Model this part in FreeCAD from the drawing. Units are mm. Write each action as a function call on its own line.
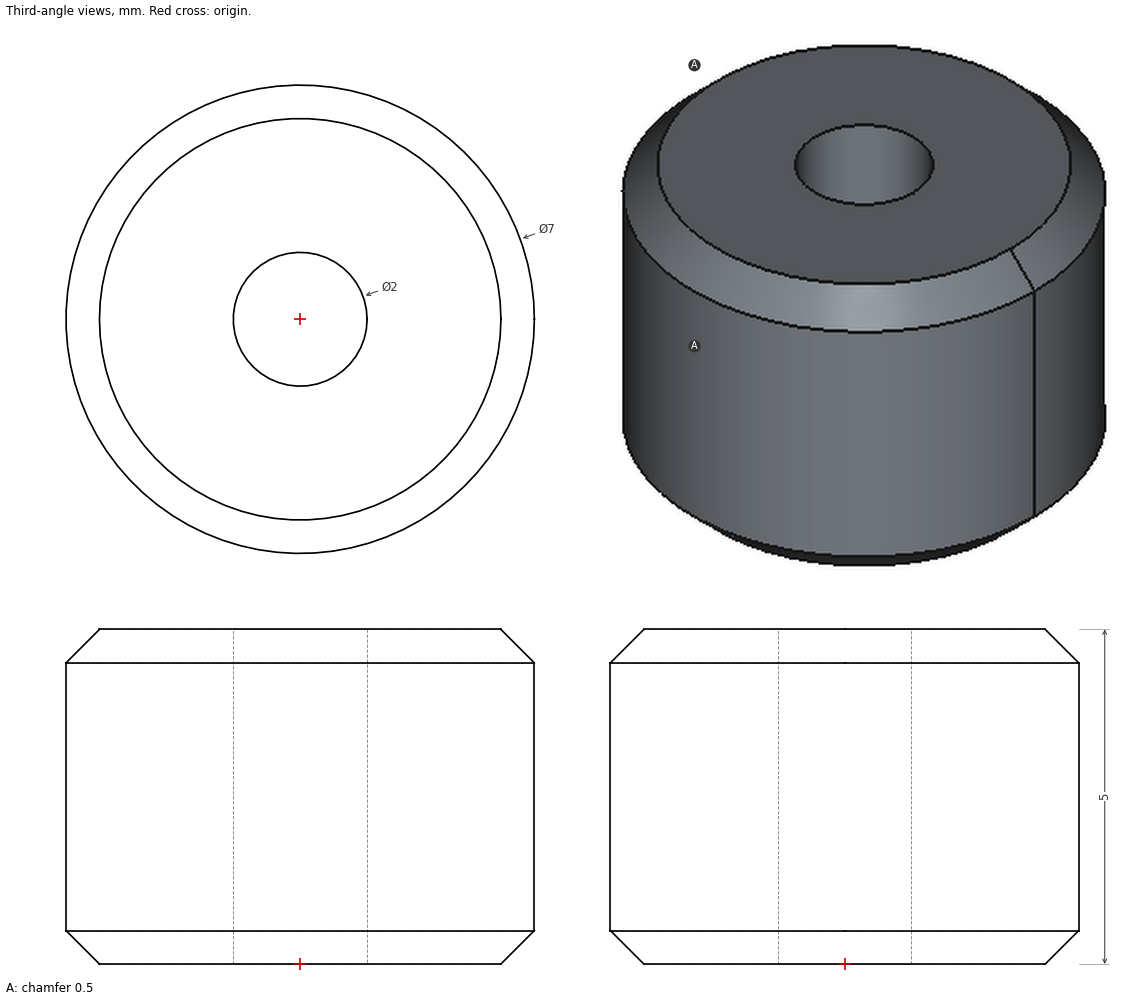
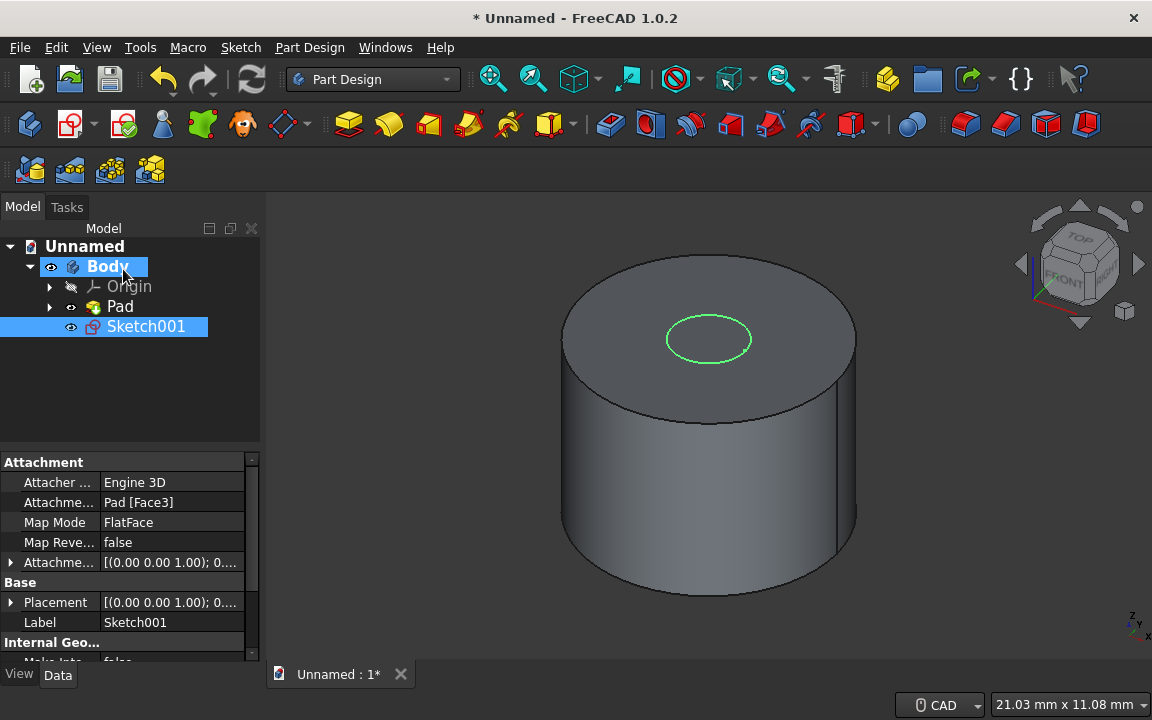
click(612, 124)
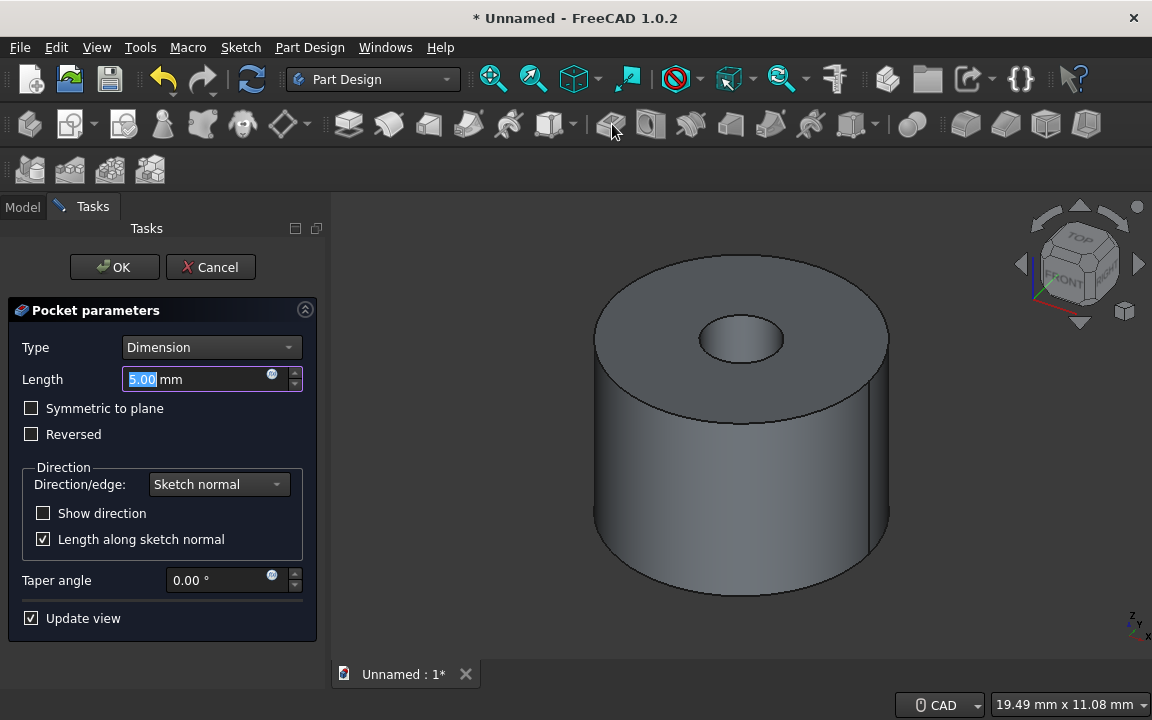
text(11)
key(Tab)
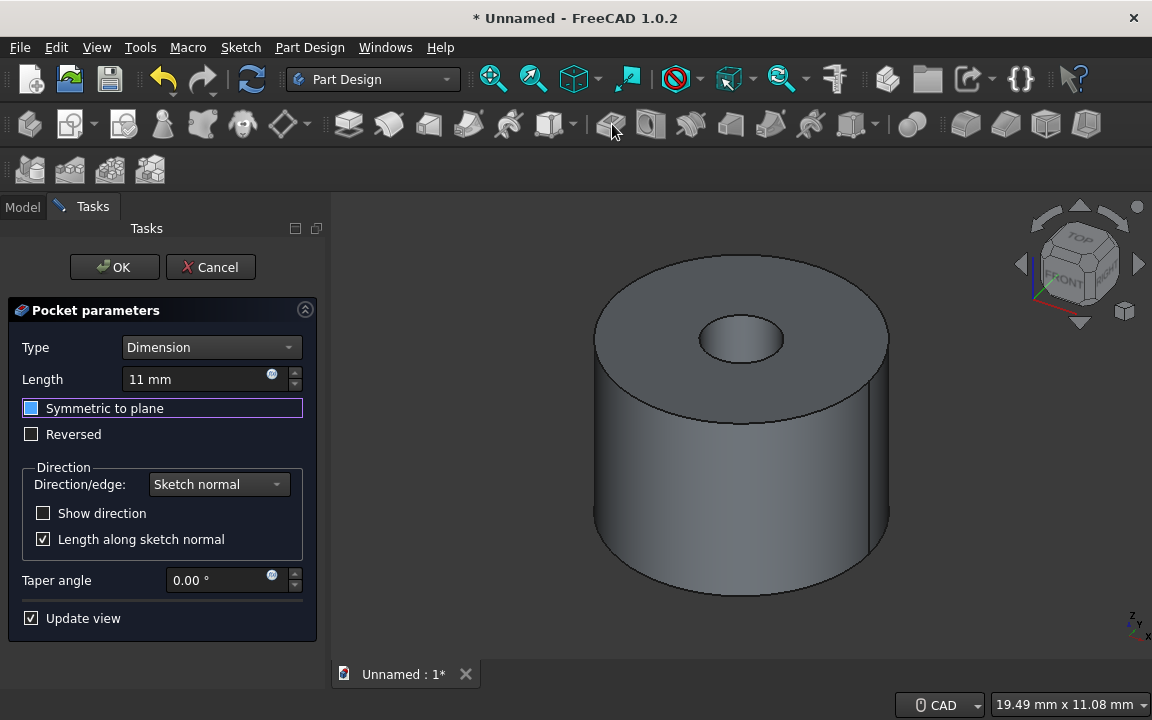
click(115, 267)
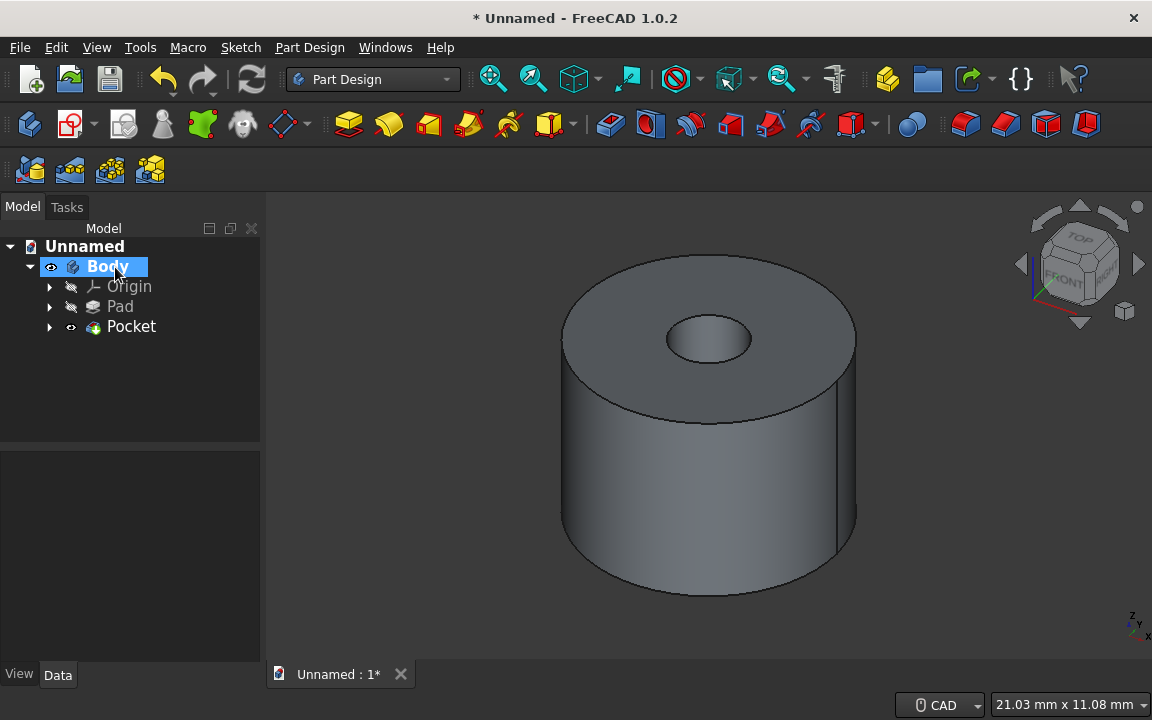
click(562, 347)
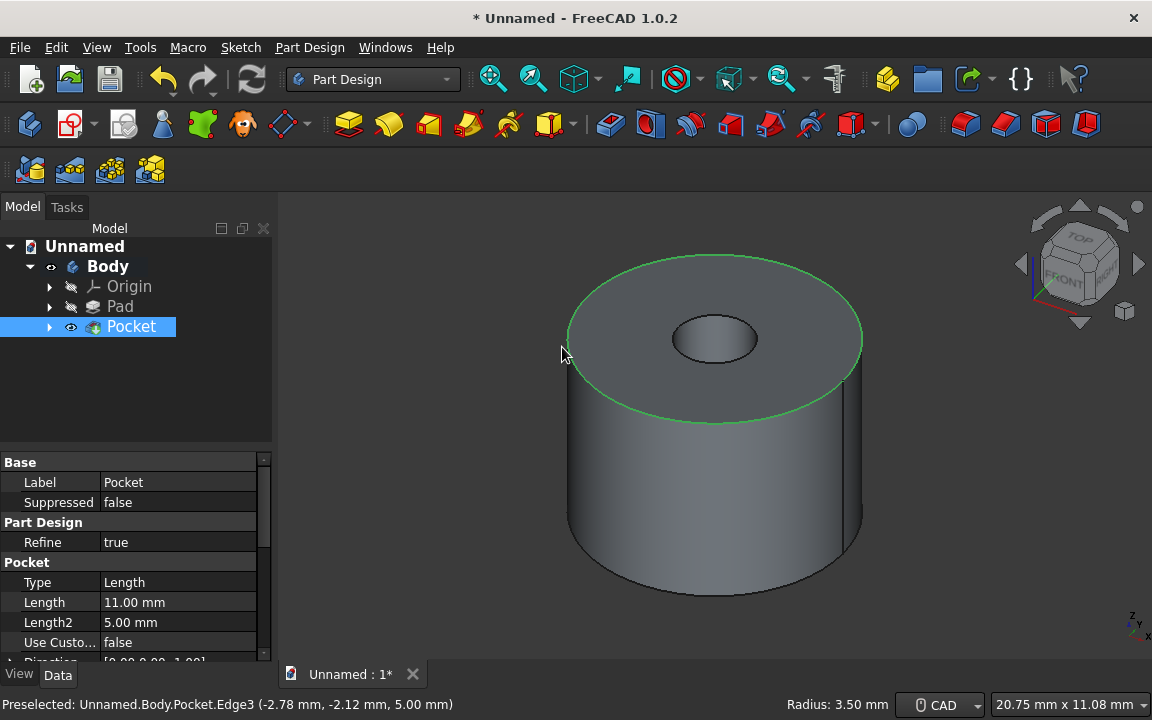
key(0)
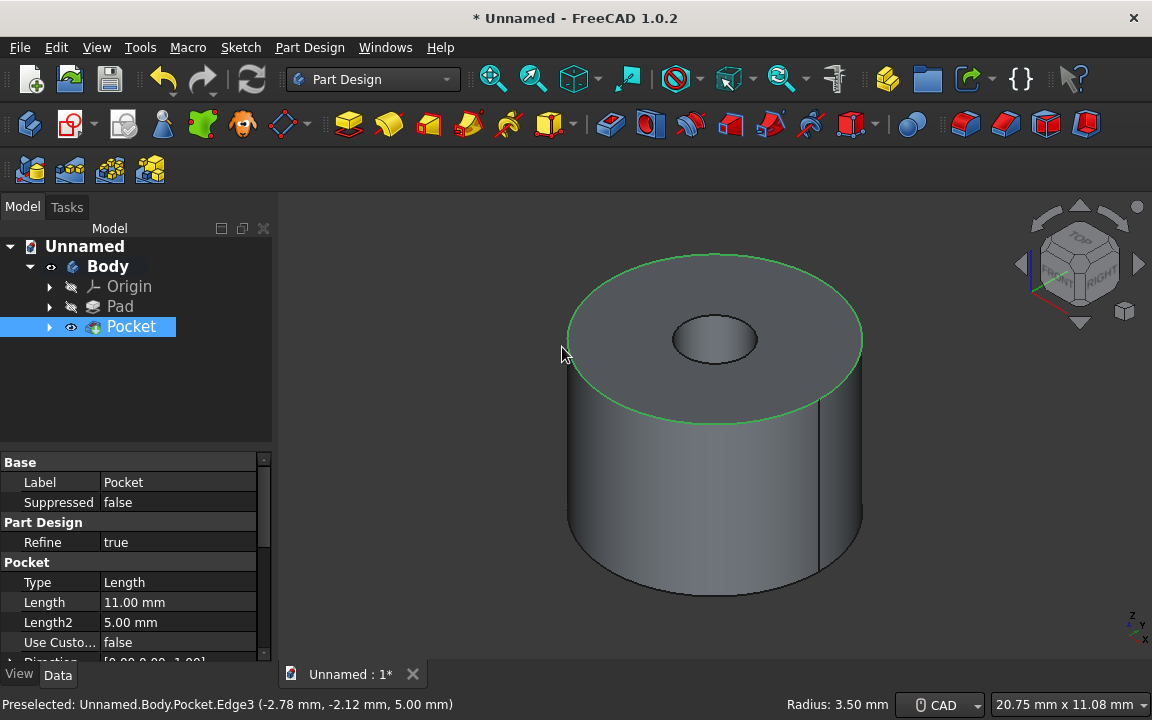
key(2)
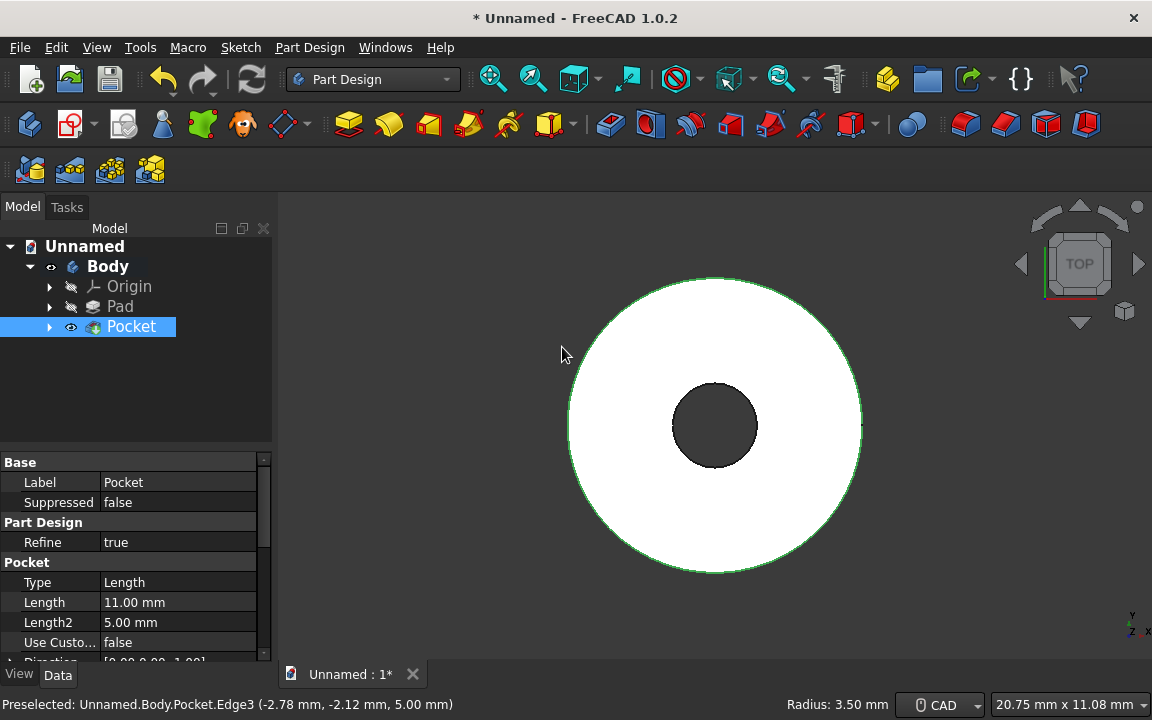
key(1)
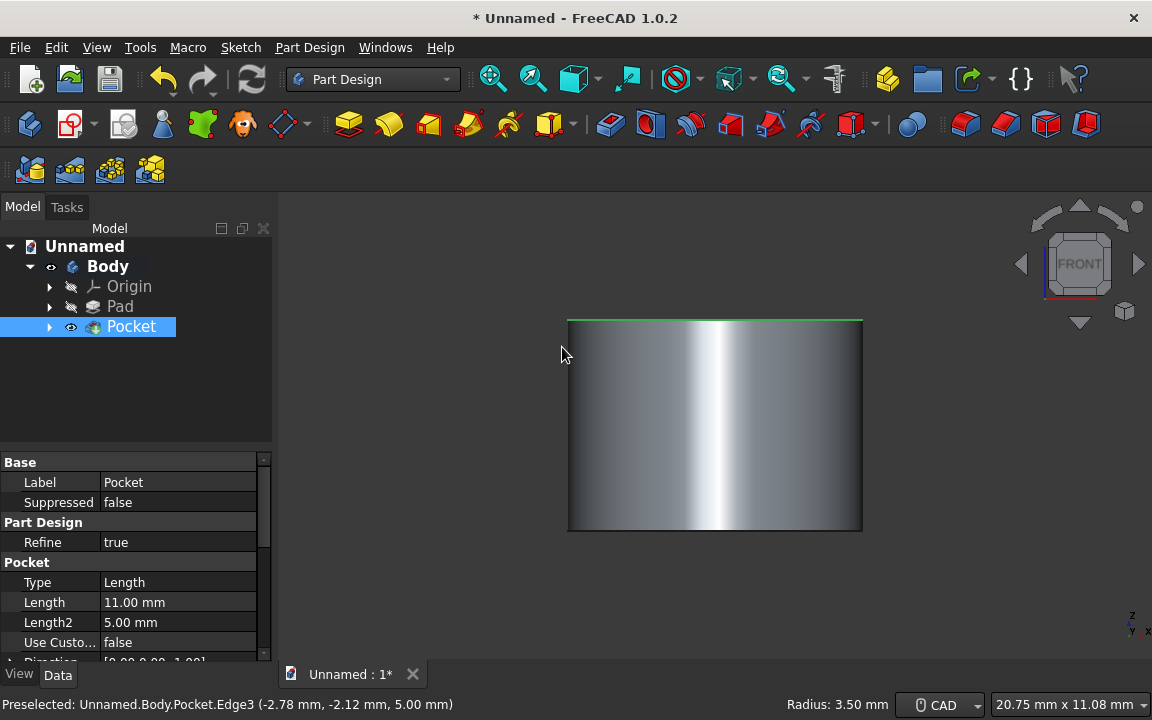
click(596, 530, ctrl)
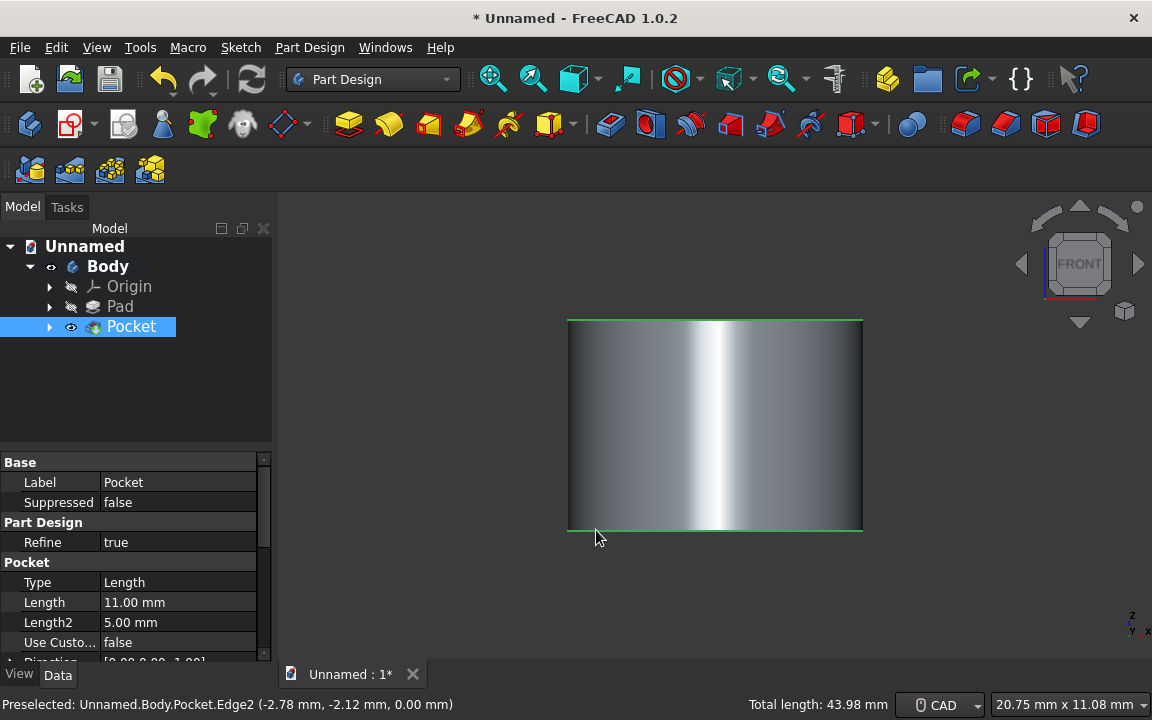
click(1006, 124)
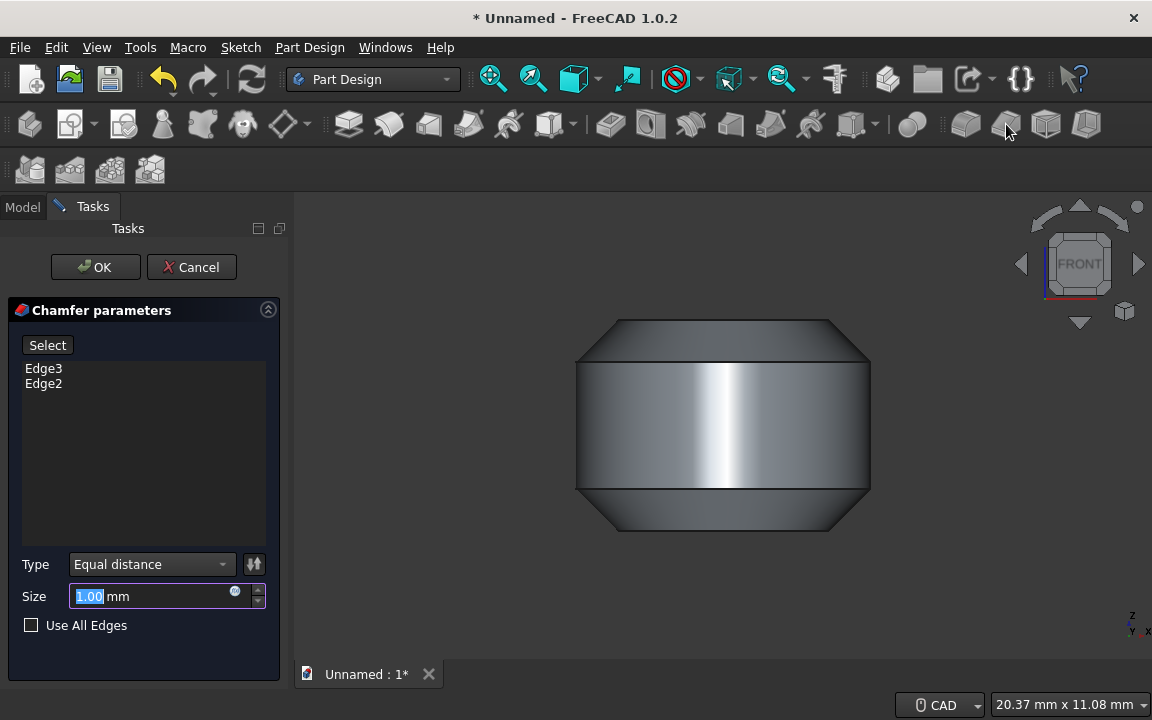
text(0.5)
key(Tab)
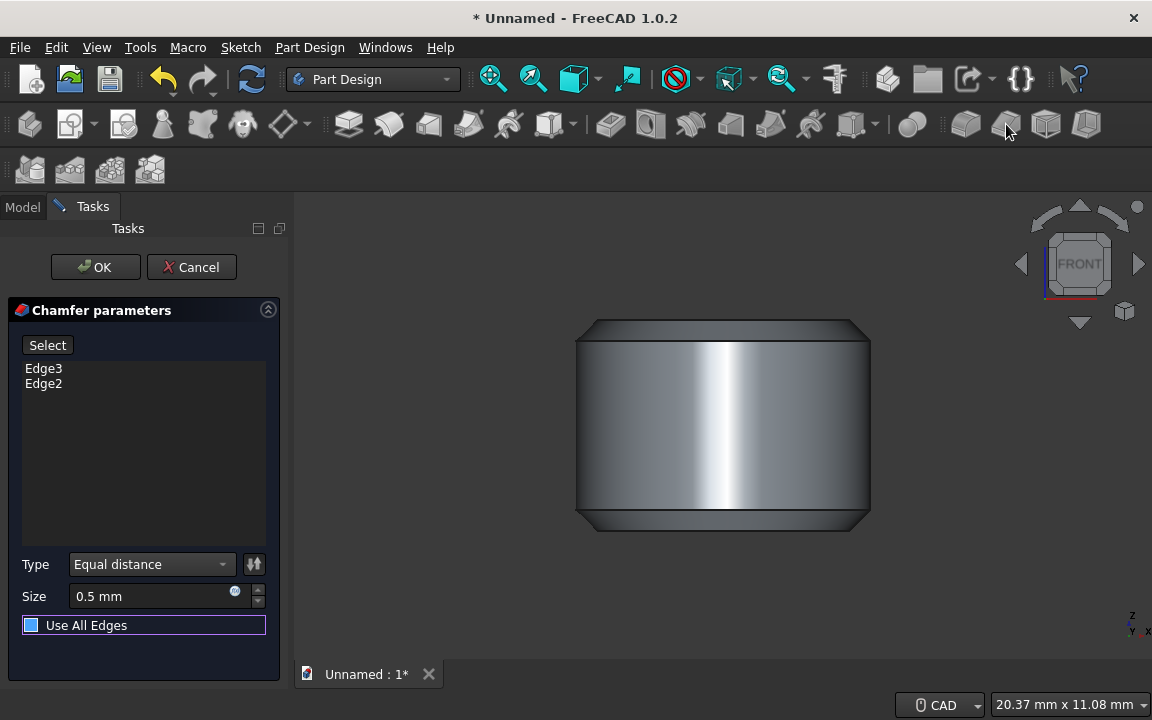
click(96, 267)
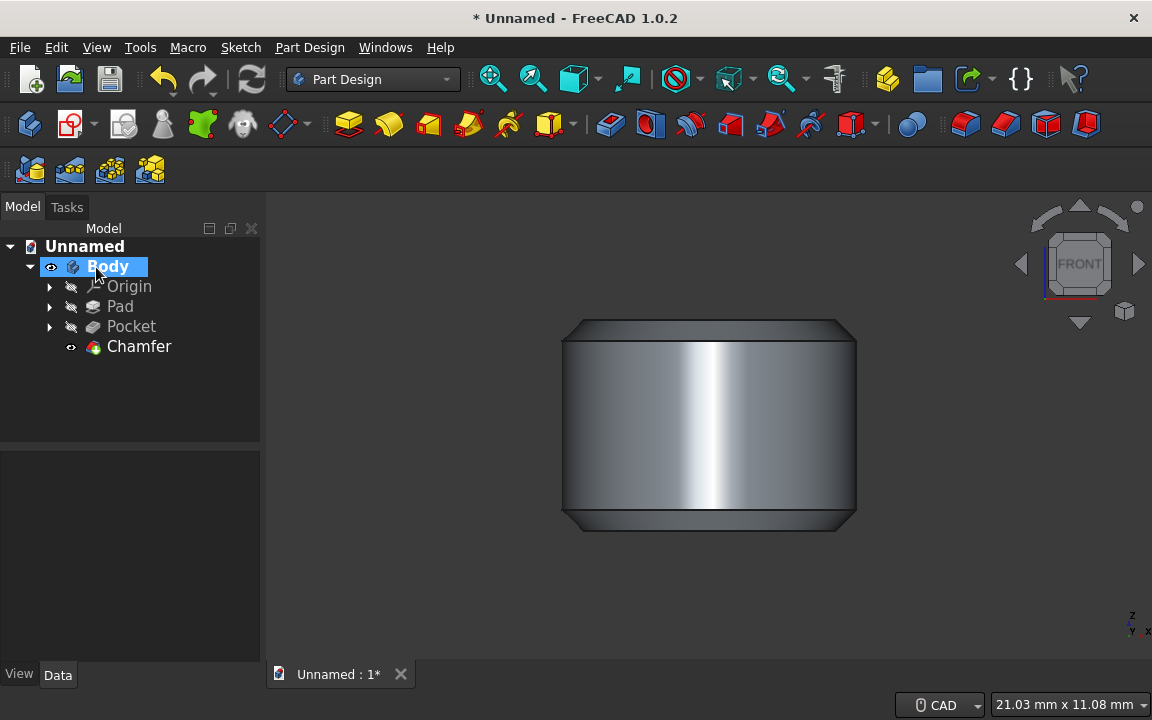
key(0)